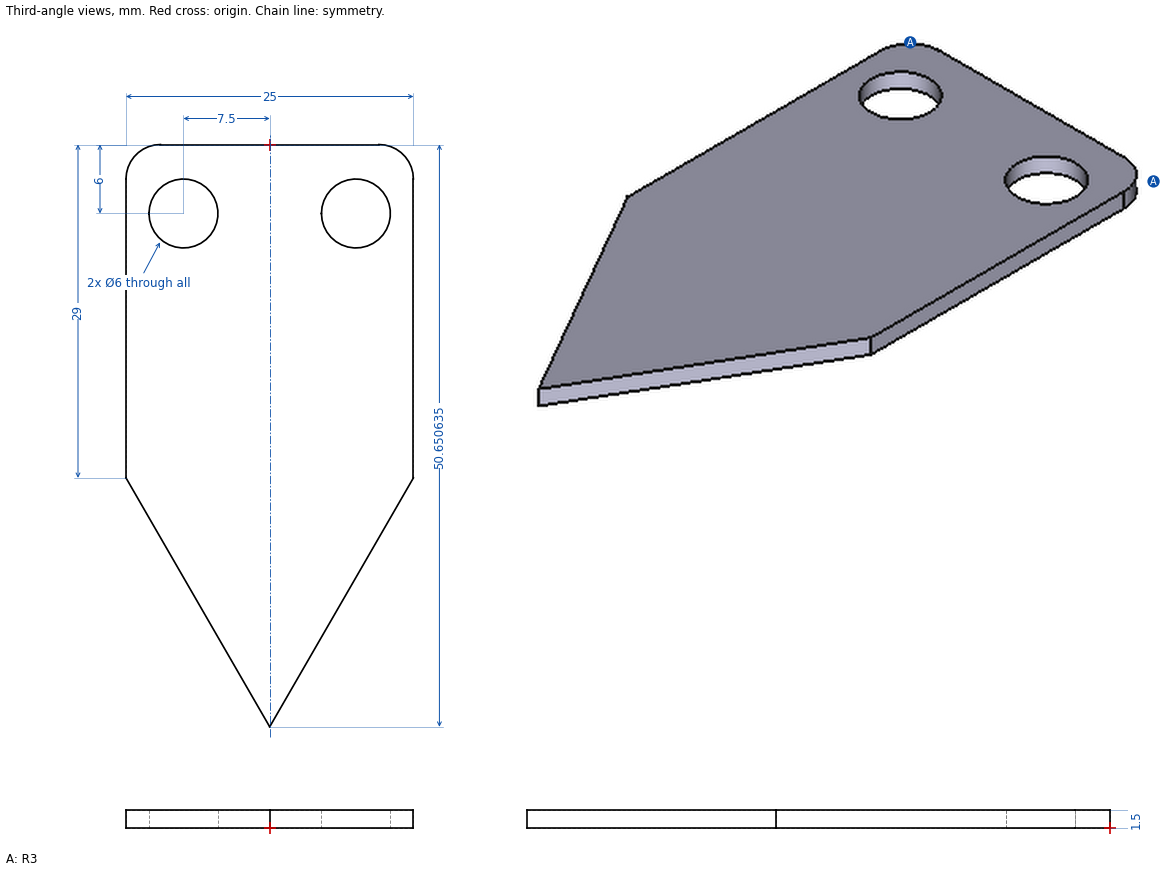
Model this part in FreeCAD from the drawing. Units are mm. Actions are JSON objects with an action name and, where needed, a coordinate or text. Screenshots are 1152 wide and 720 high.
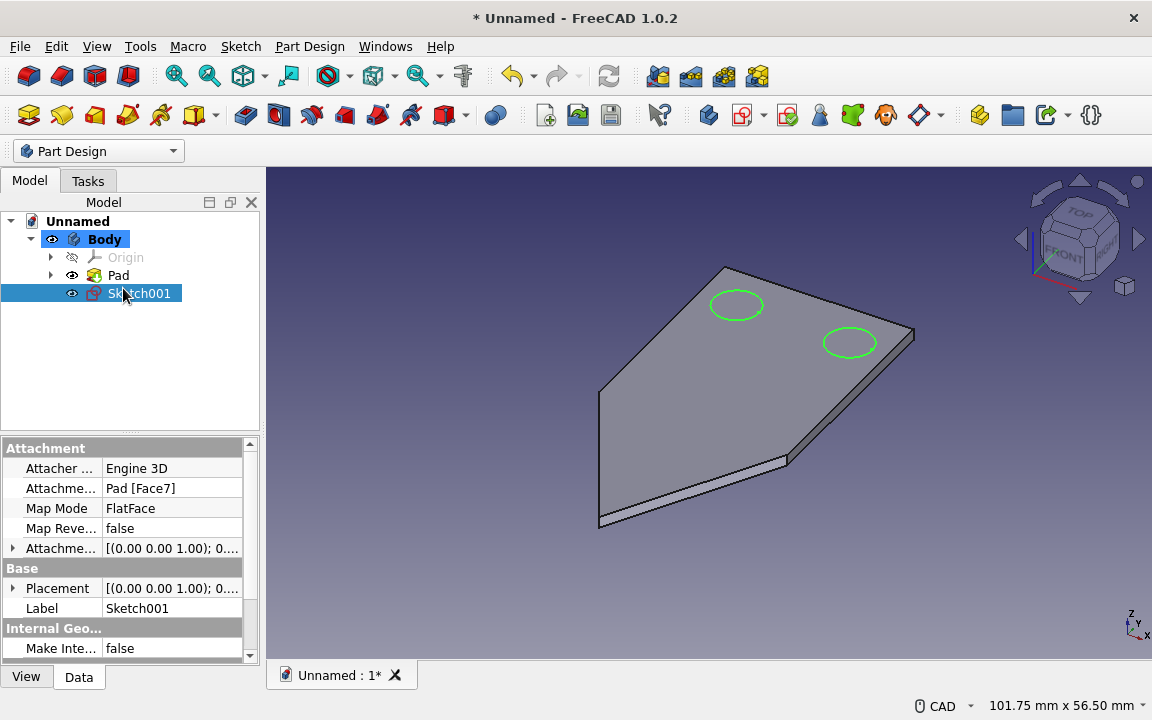
{"action": "left_click", "coordinate": [279, 116]}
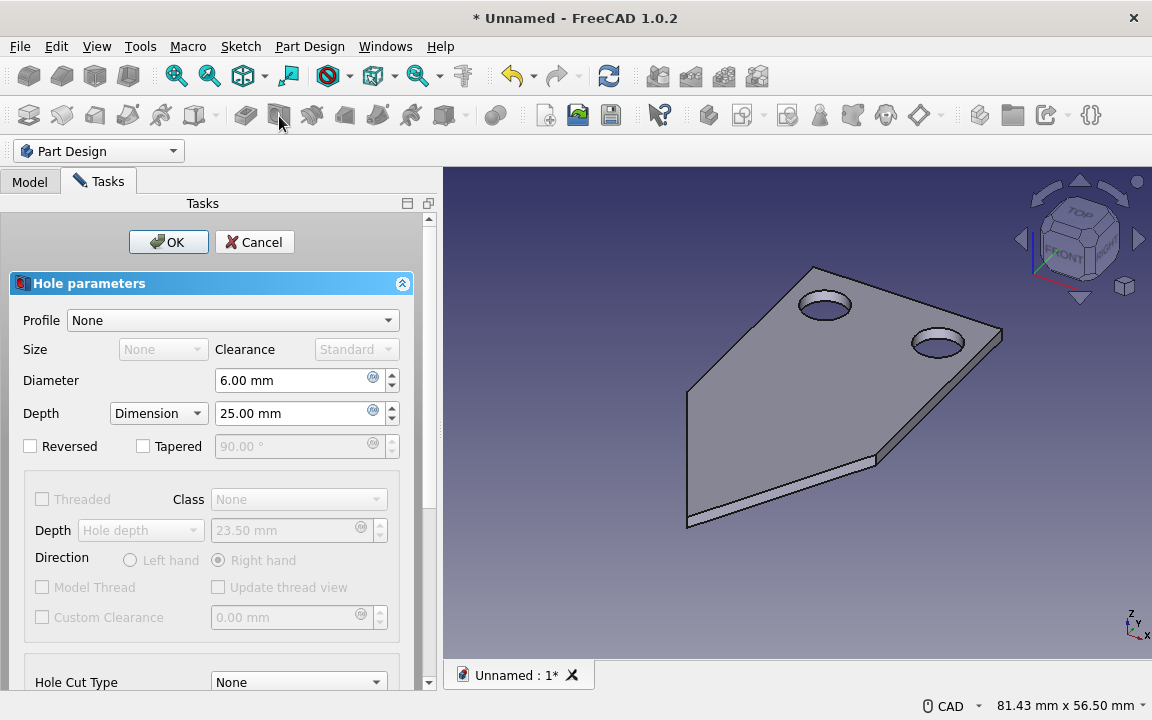
{"action": "triple_click", "coordinate": [300, 380]}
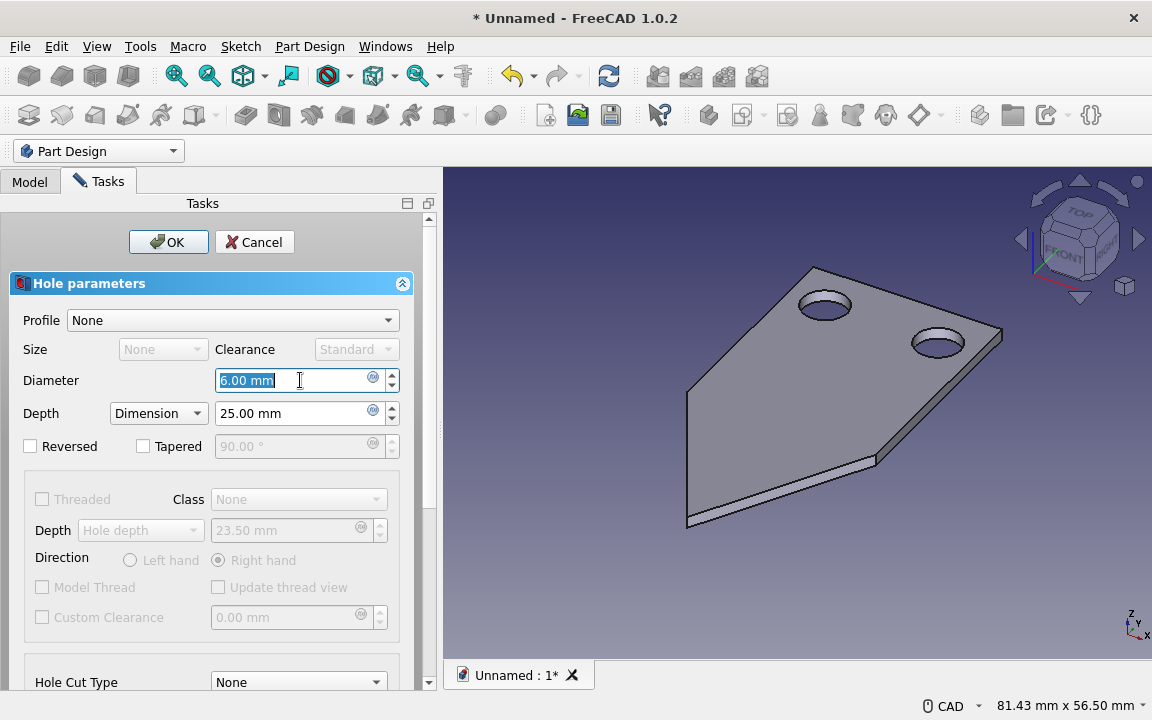
{"action": "type", "text": "6"}
{"action": "key", "text": "Tab"}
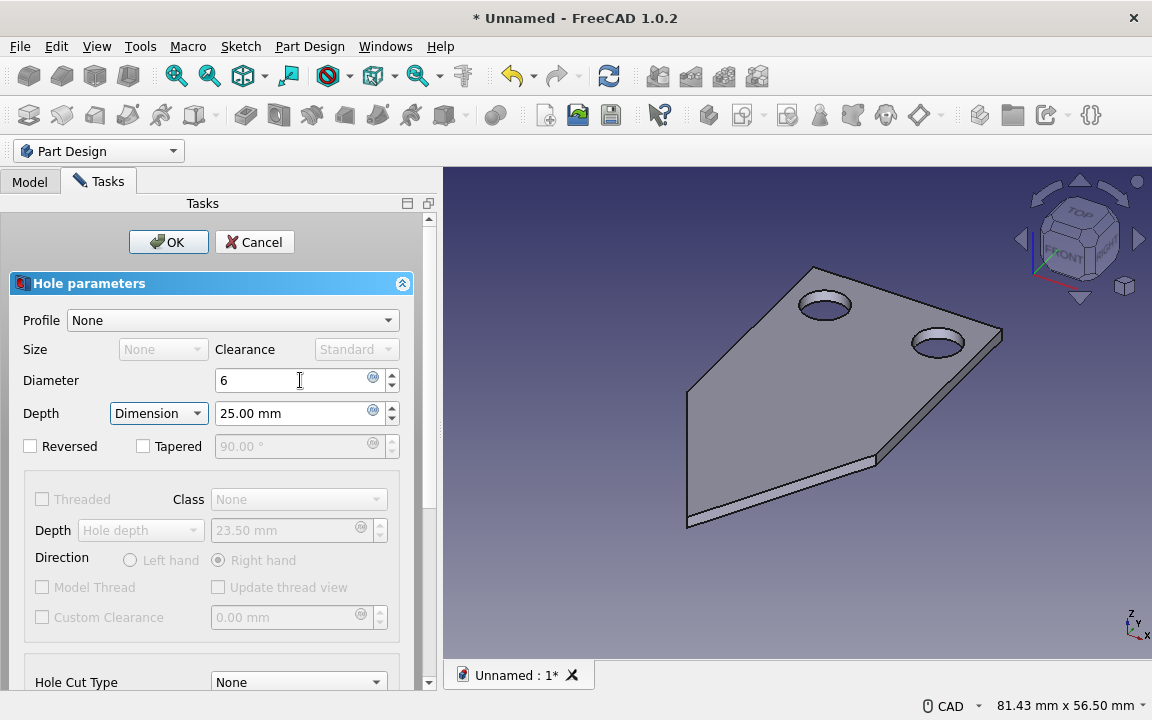
{"action": "left_click", "coordinate": [160, 414]}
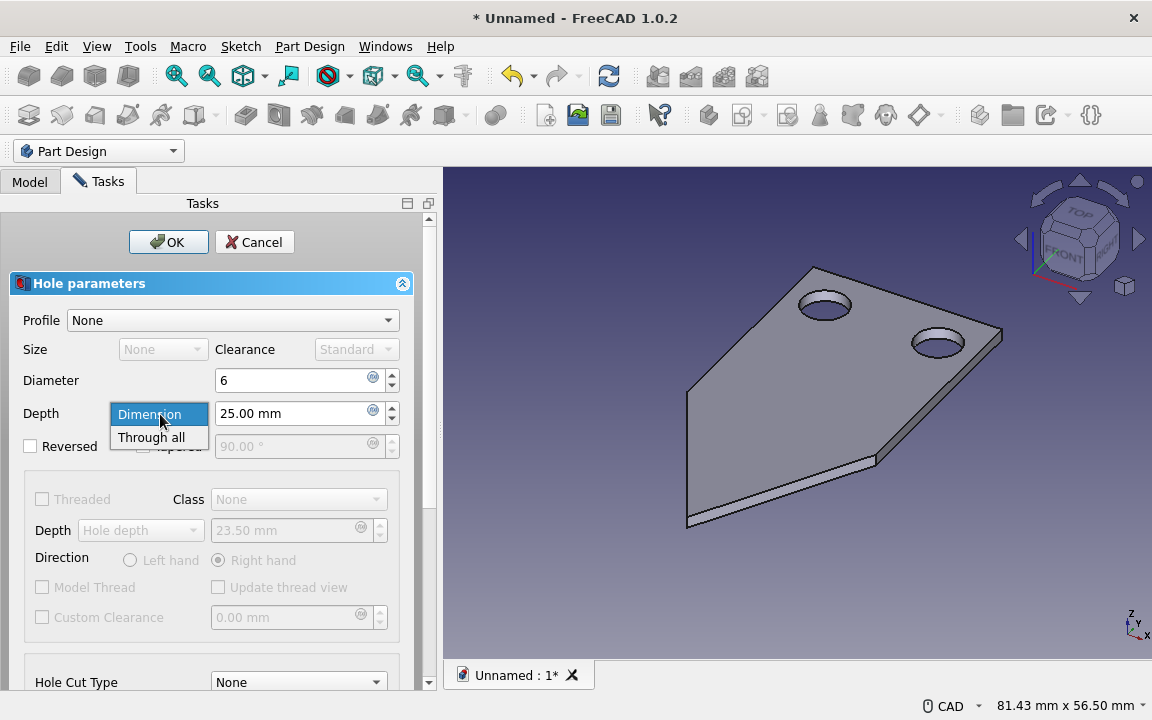
{"action": "left_click", "coordinate": [158, 438]}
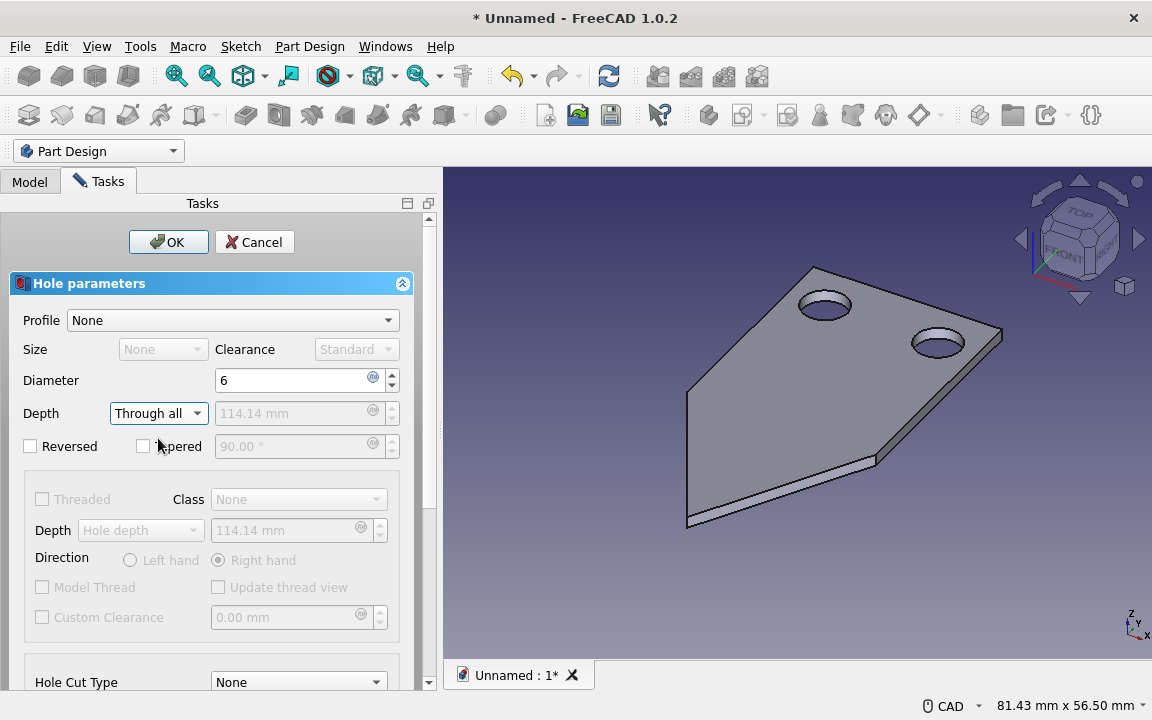
{"action": "left_click", "coordinate": [169, 242]}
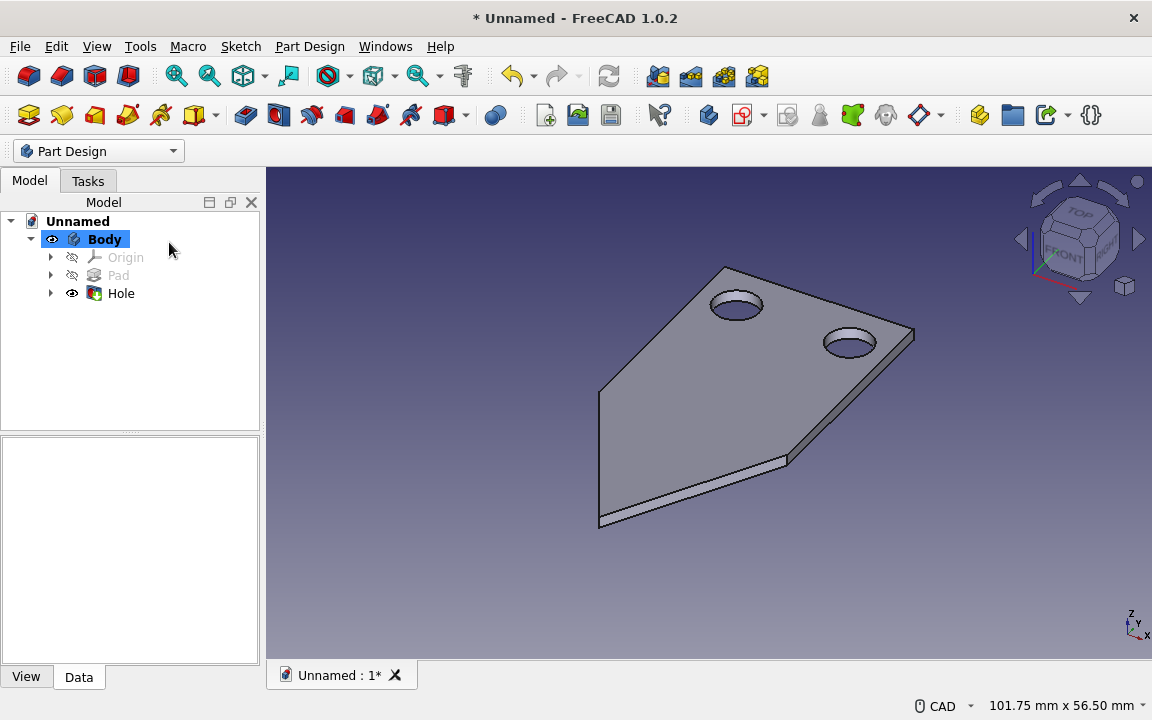
{"action": "scroll", "coordinate": [725, 271], "scroll_direction": "up", "scroll_amount": 6}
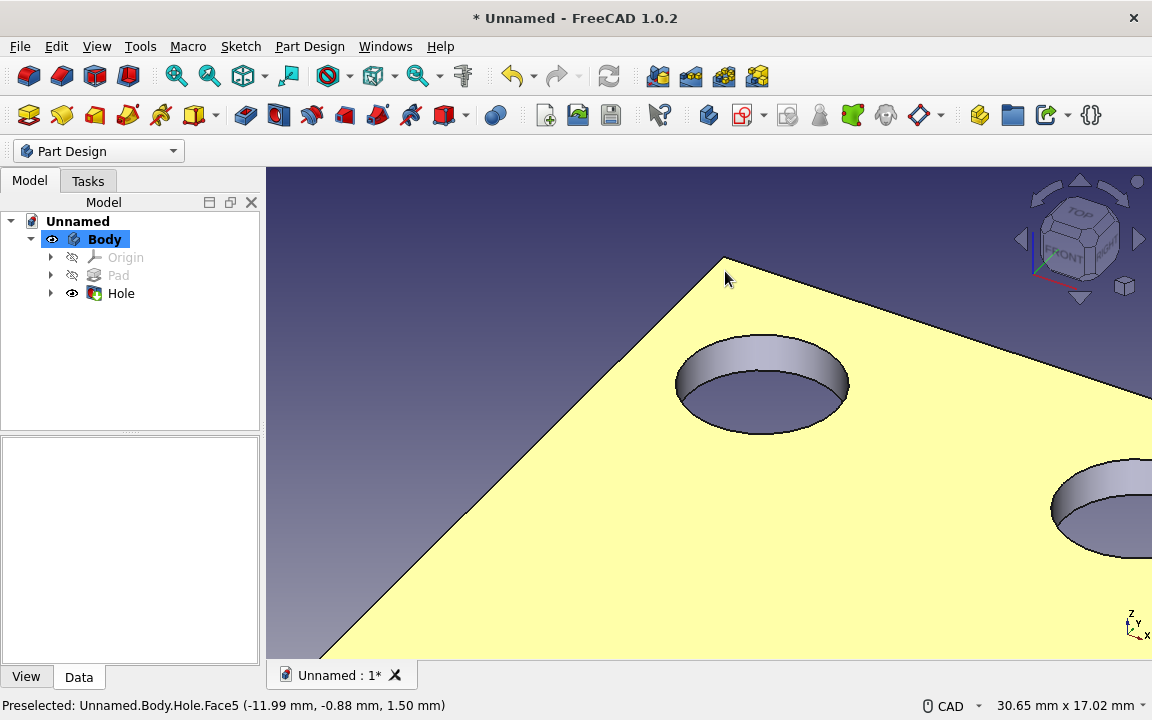
{"action": "left_click", "coordinate": [177, 76]}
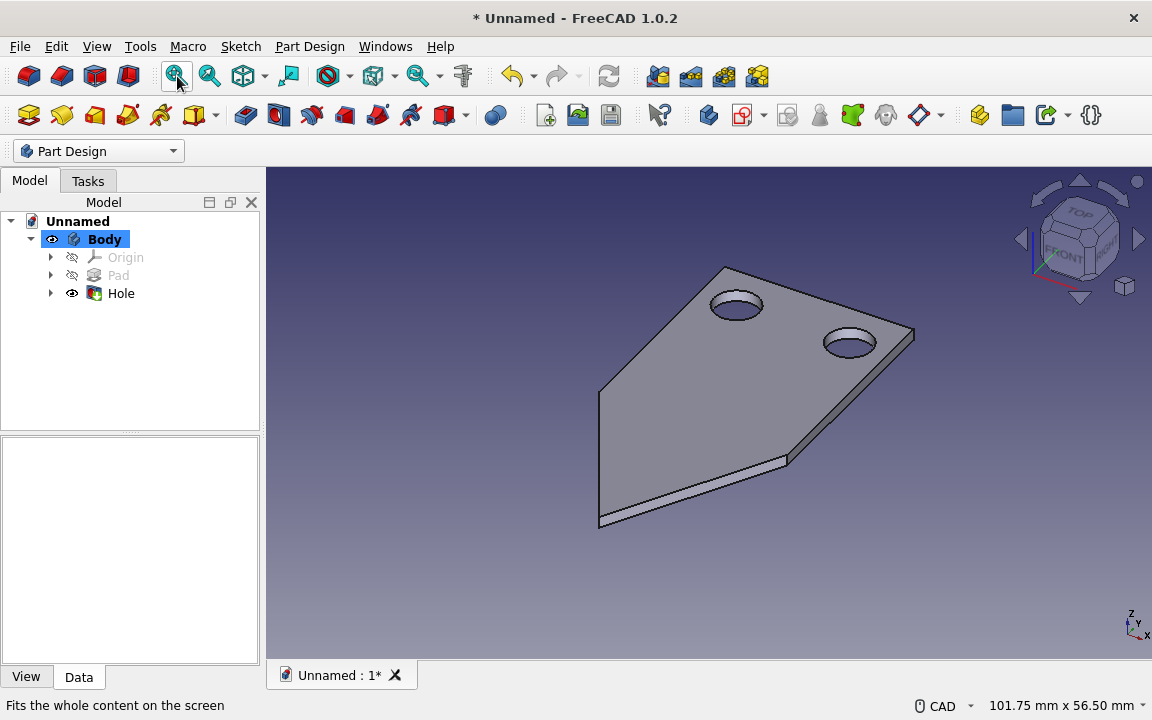
{"action": "key", "text": "0"}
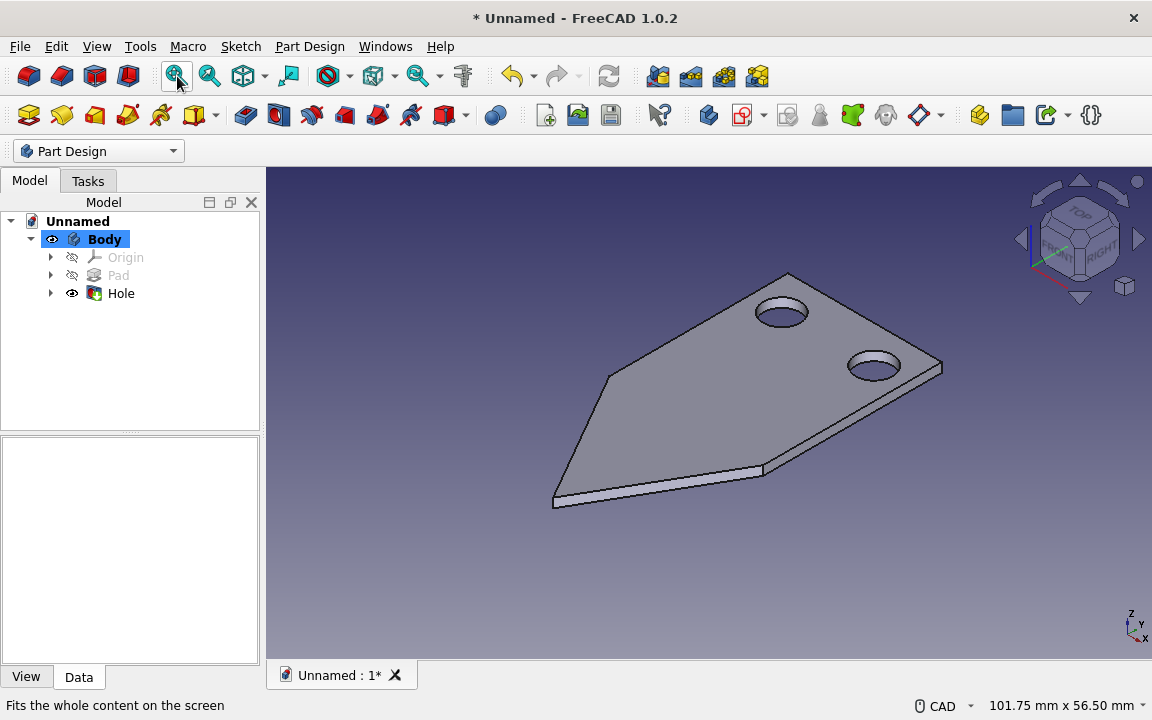
{"action": "scroll", "coordinate": [788, 278], "scroll_direction": "up", "scroll_amount": 6}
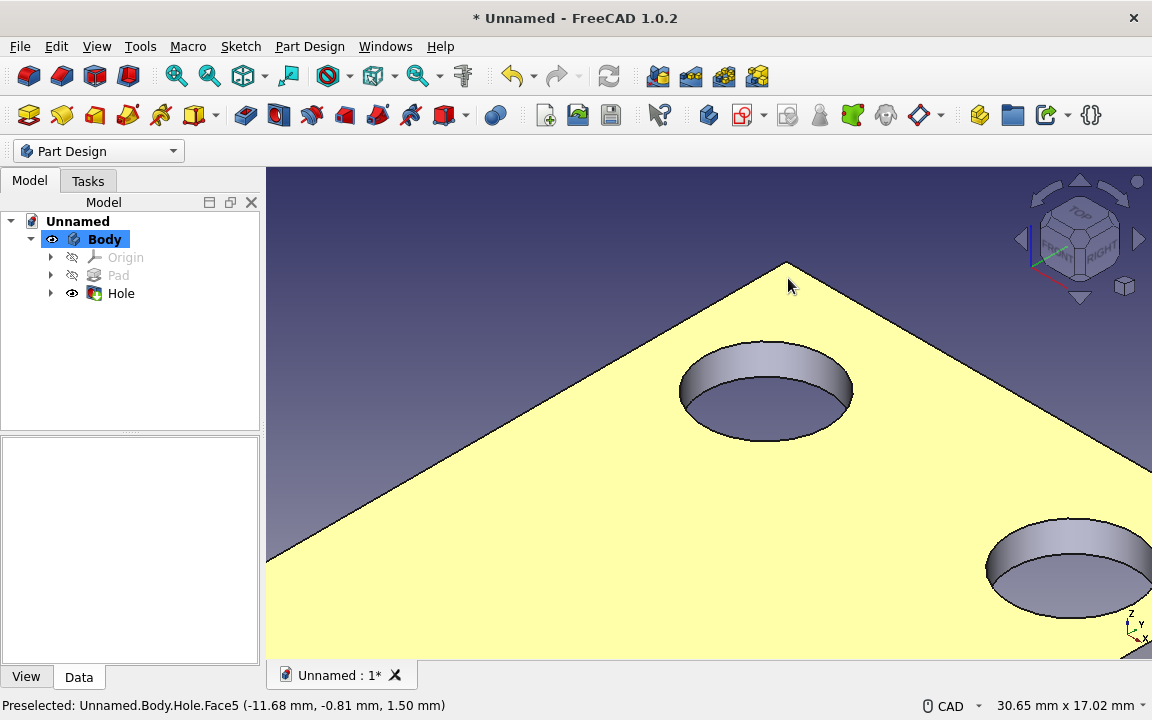
{"action": "left_click", "coordinate": [177, 76]}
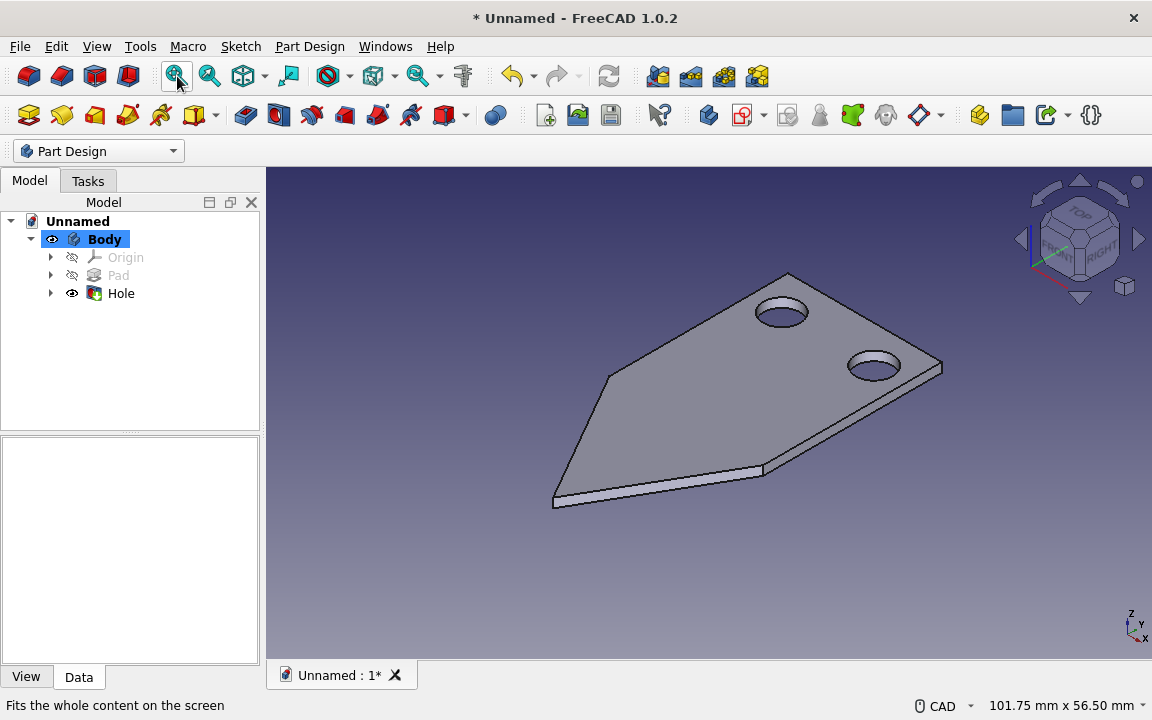
{"action": "key", "text": "2"}